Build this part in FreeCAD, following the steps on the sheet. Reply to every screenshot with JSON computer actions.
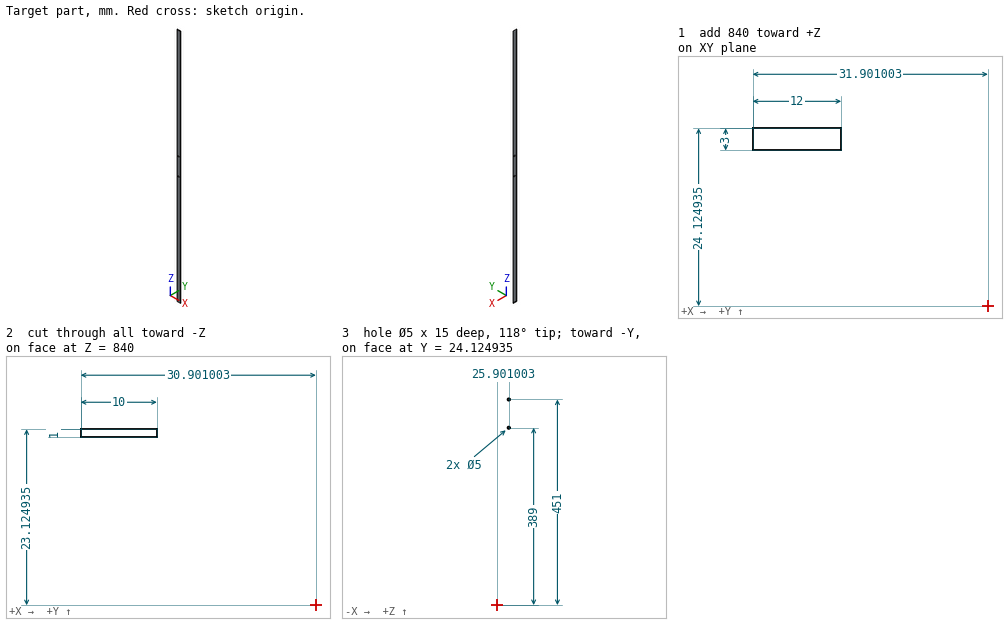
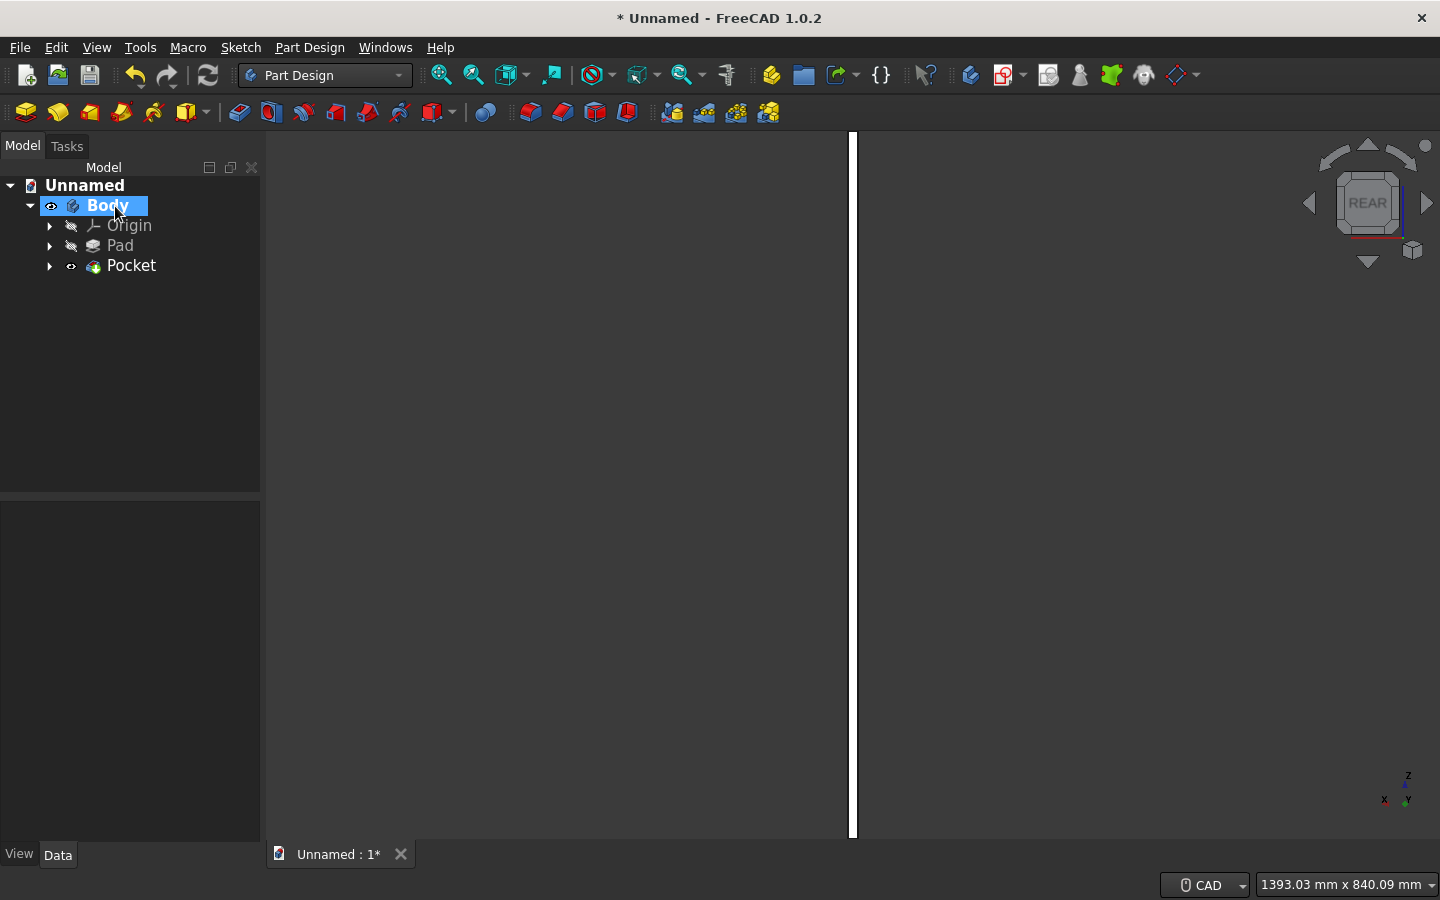
{"action": "left_click", "coordinate": [442, 76]}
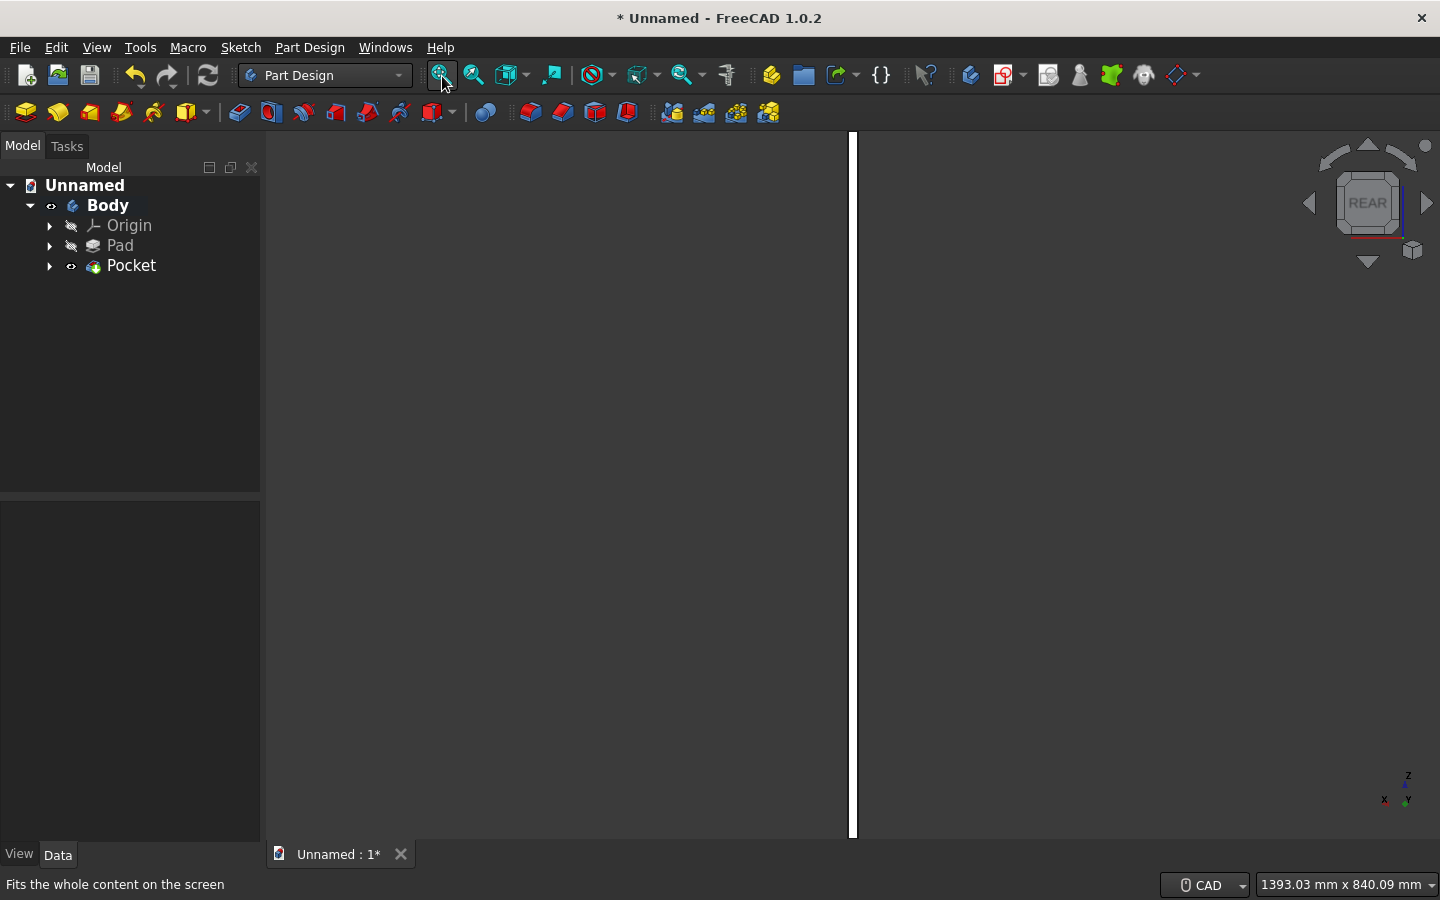
{"action": "scroll", "coordinate": [853, 181], "scroll_direction": "up", "scroll_amount": 5}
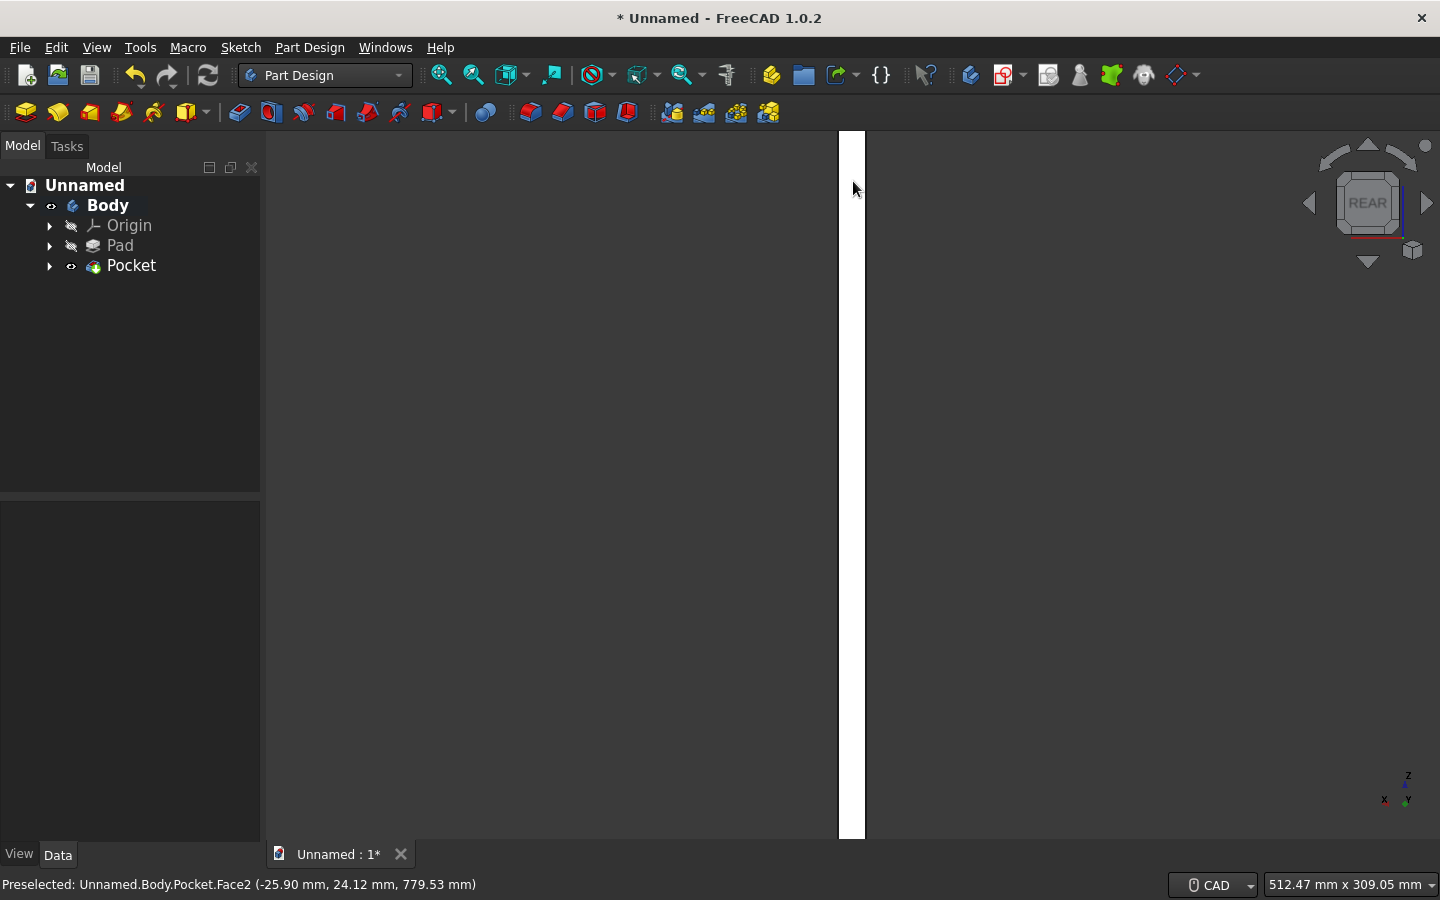
{"action": "left_click", "coordinate": [852, 182]}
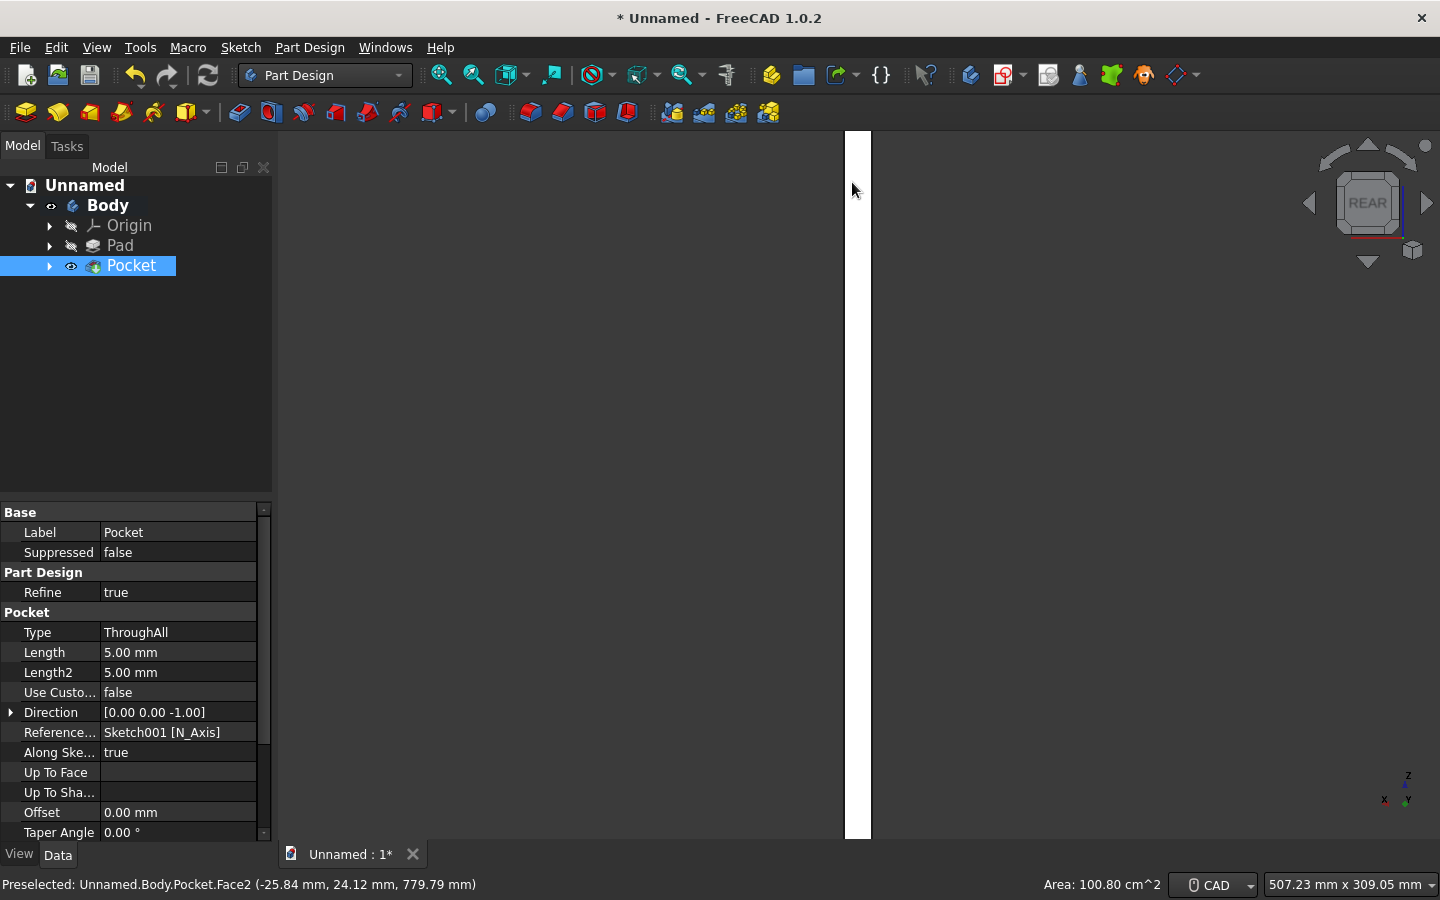
{"action": "left_click", "coordinate": [1004, 76]}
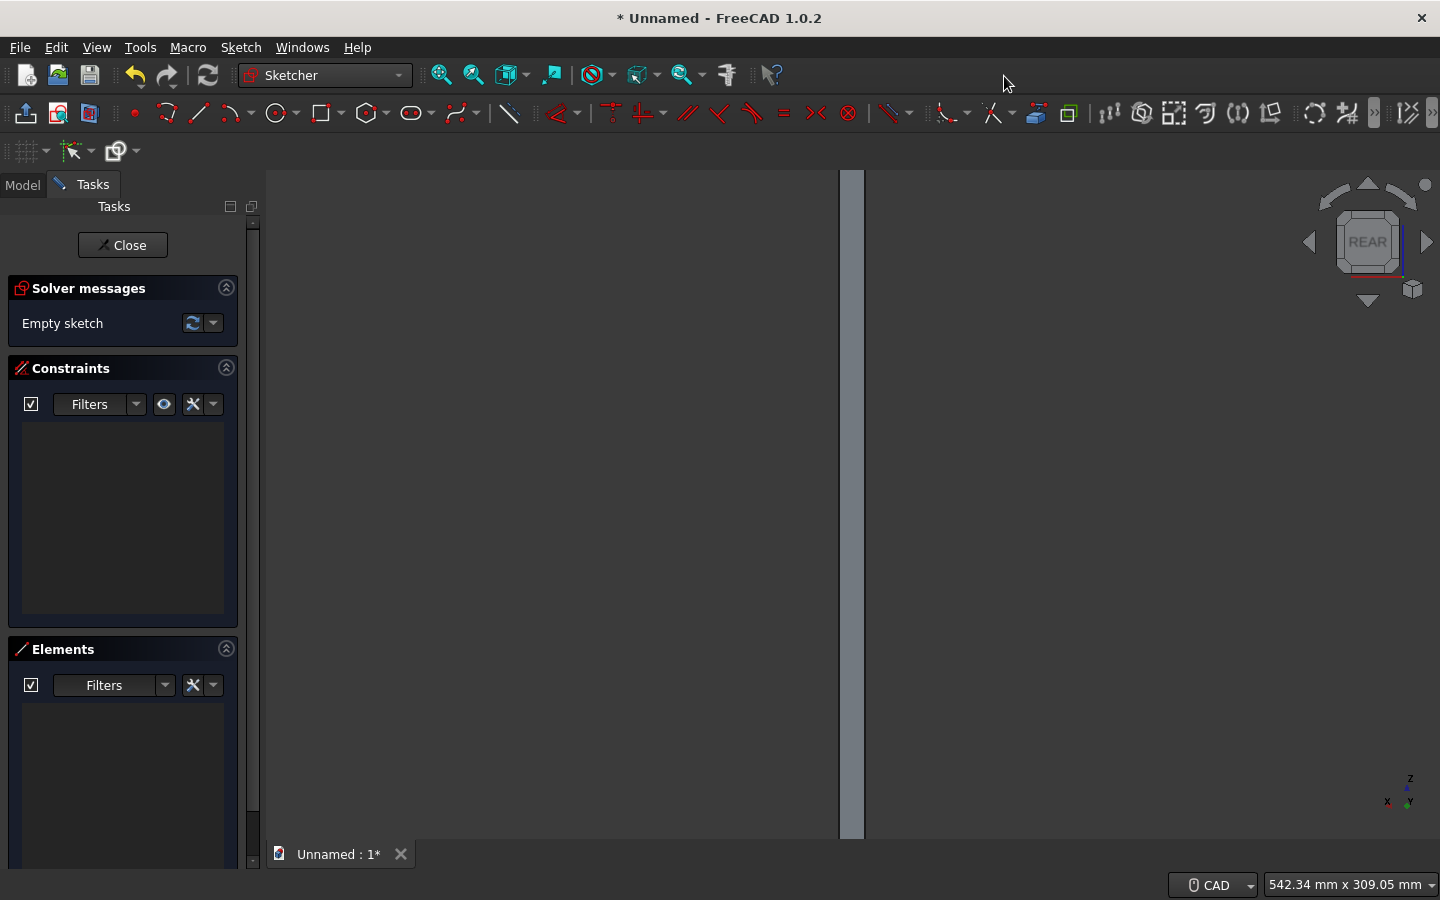
{"action": "scroll", "coordinate": [784, 504], "scroll_direction": "down", "scroll_amount": 5}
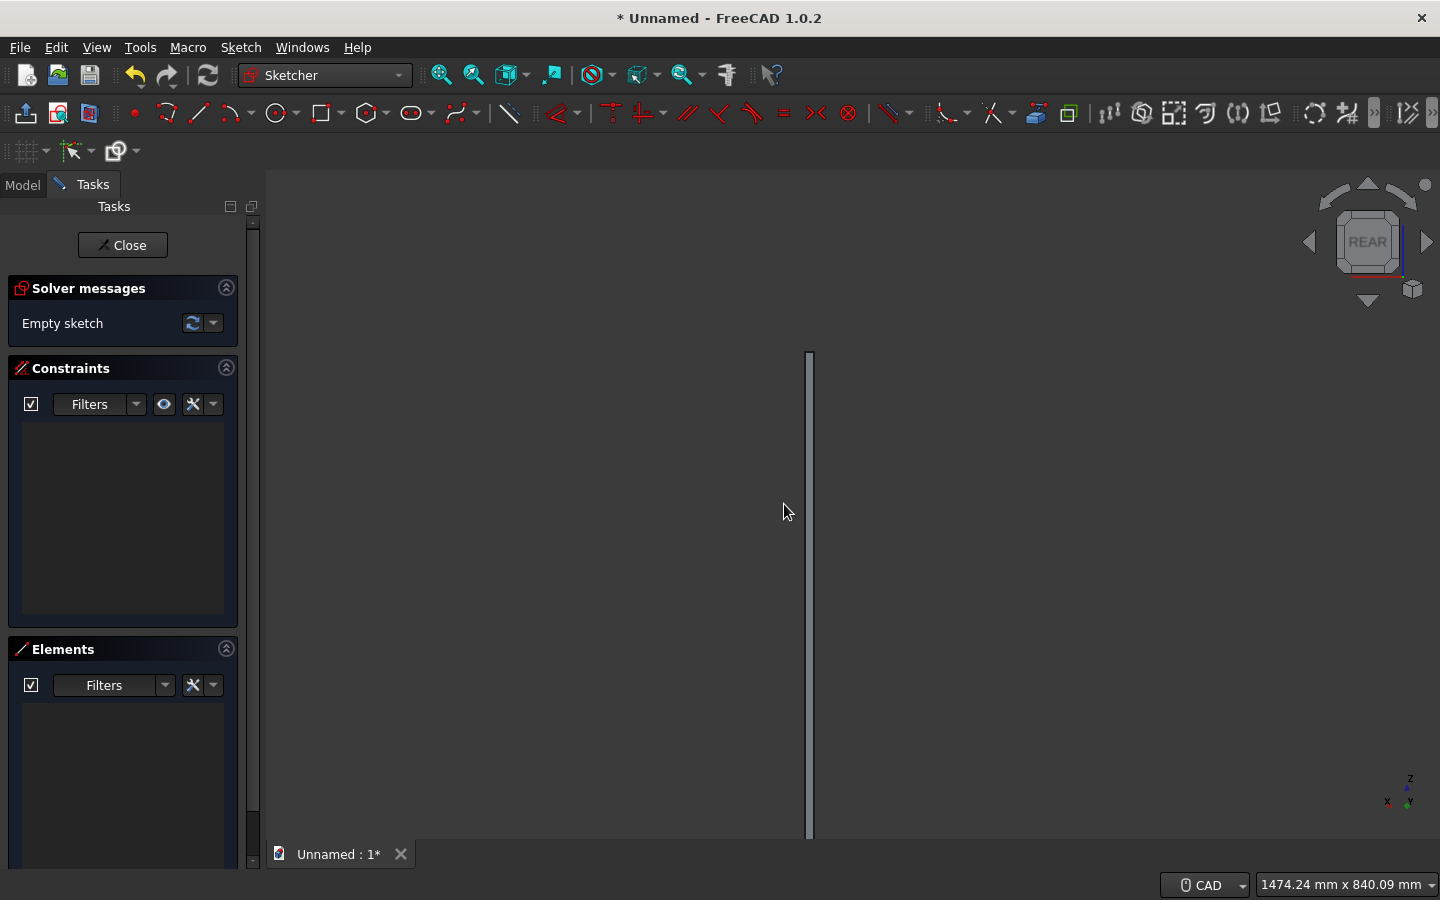
{"action": "scroll", "coordinate": [813, 714], "scroll_direction": "up", "scroll_amount": 10}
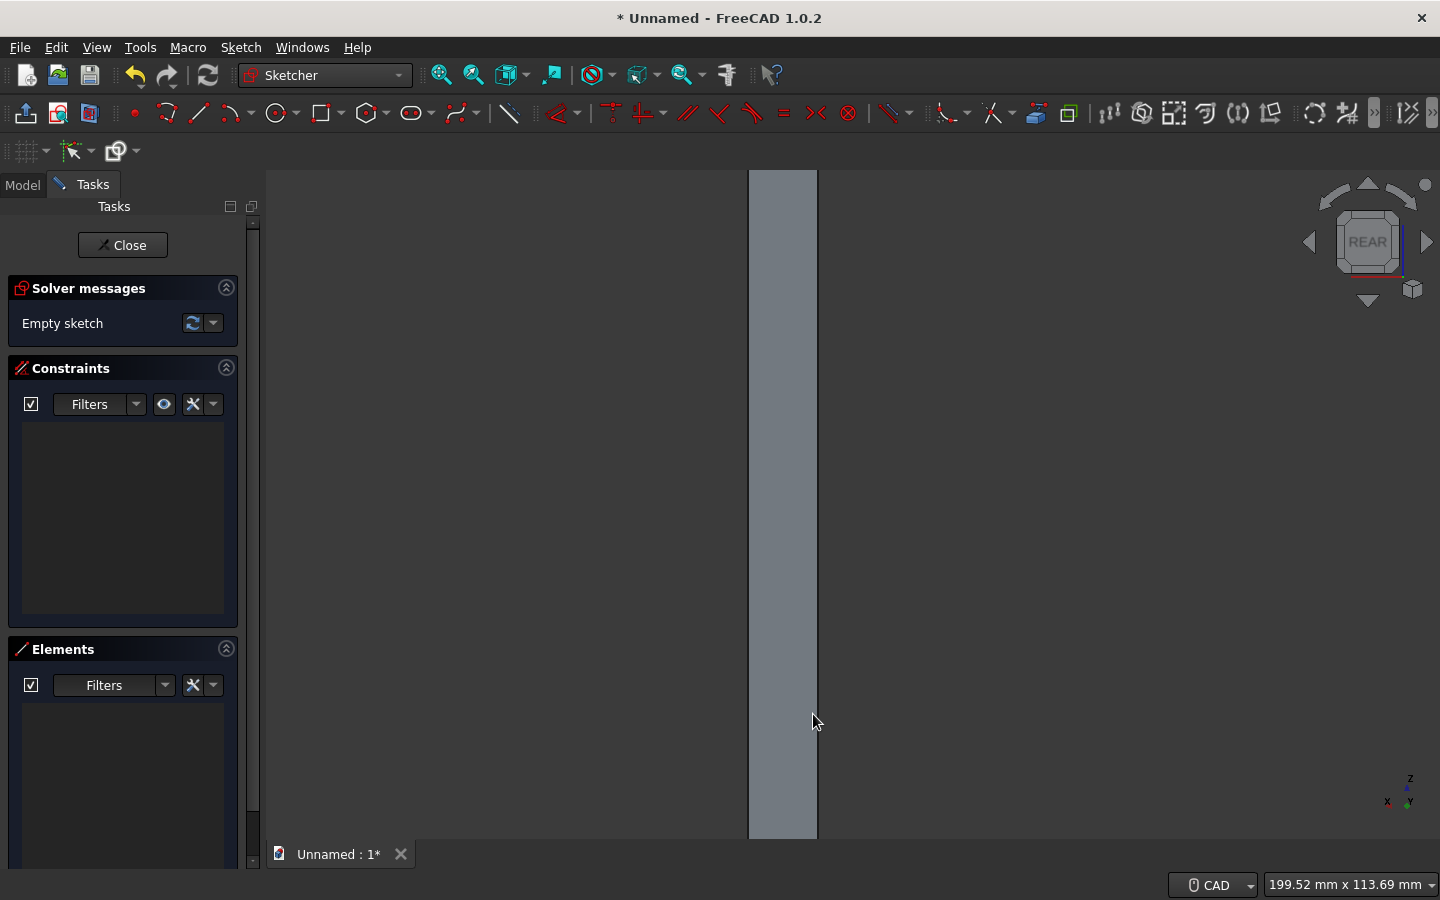
{"action": "left_click", "coordinate": [276, 114]}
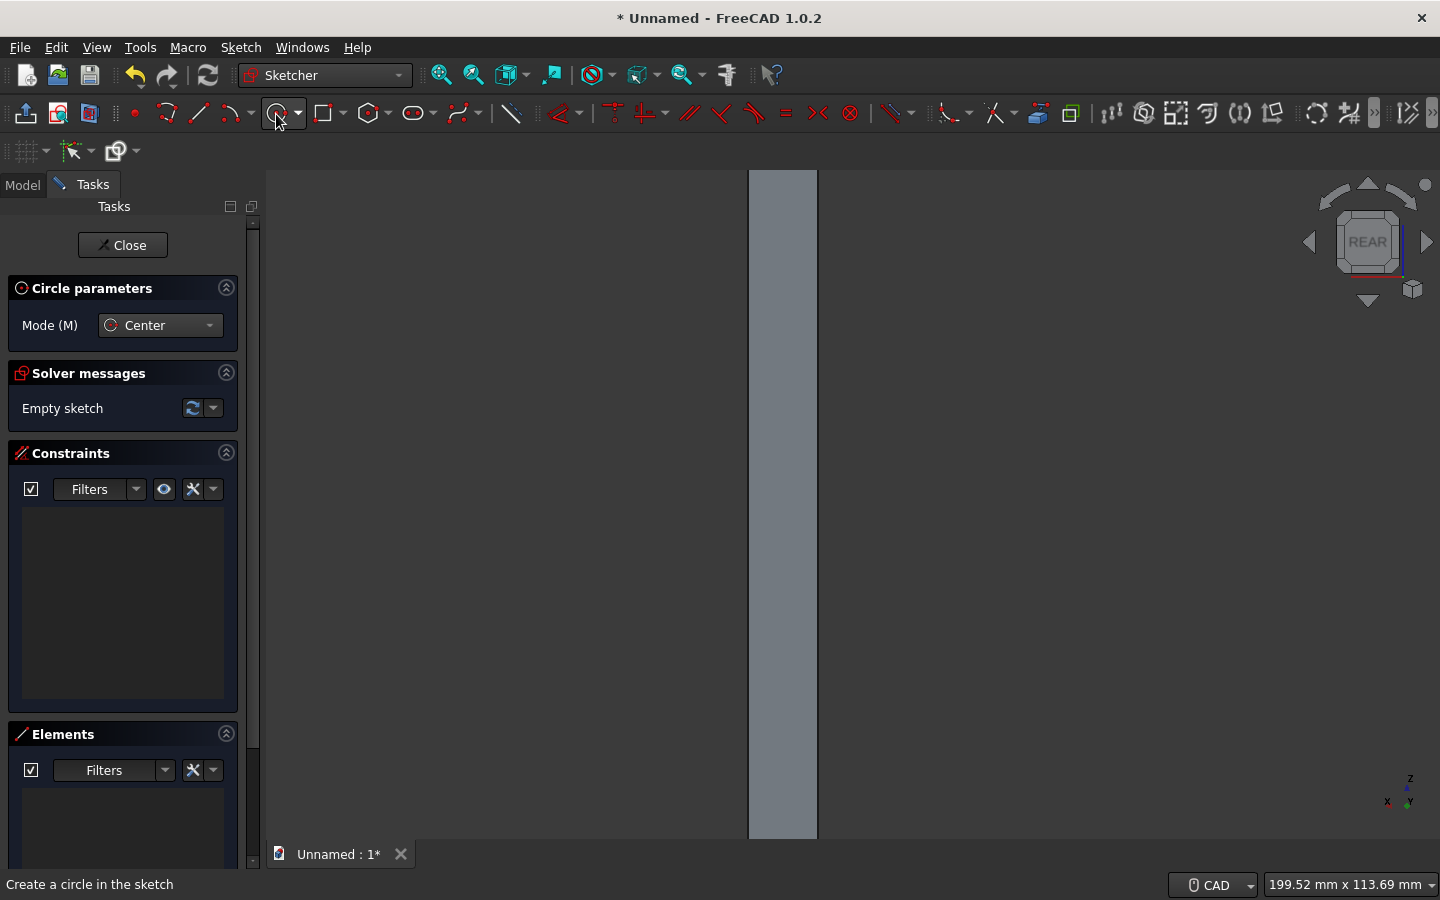
{"action": "scroll", "coordinate": [783, 685], "scroll_direction": "up", "scroll_amount": 3}